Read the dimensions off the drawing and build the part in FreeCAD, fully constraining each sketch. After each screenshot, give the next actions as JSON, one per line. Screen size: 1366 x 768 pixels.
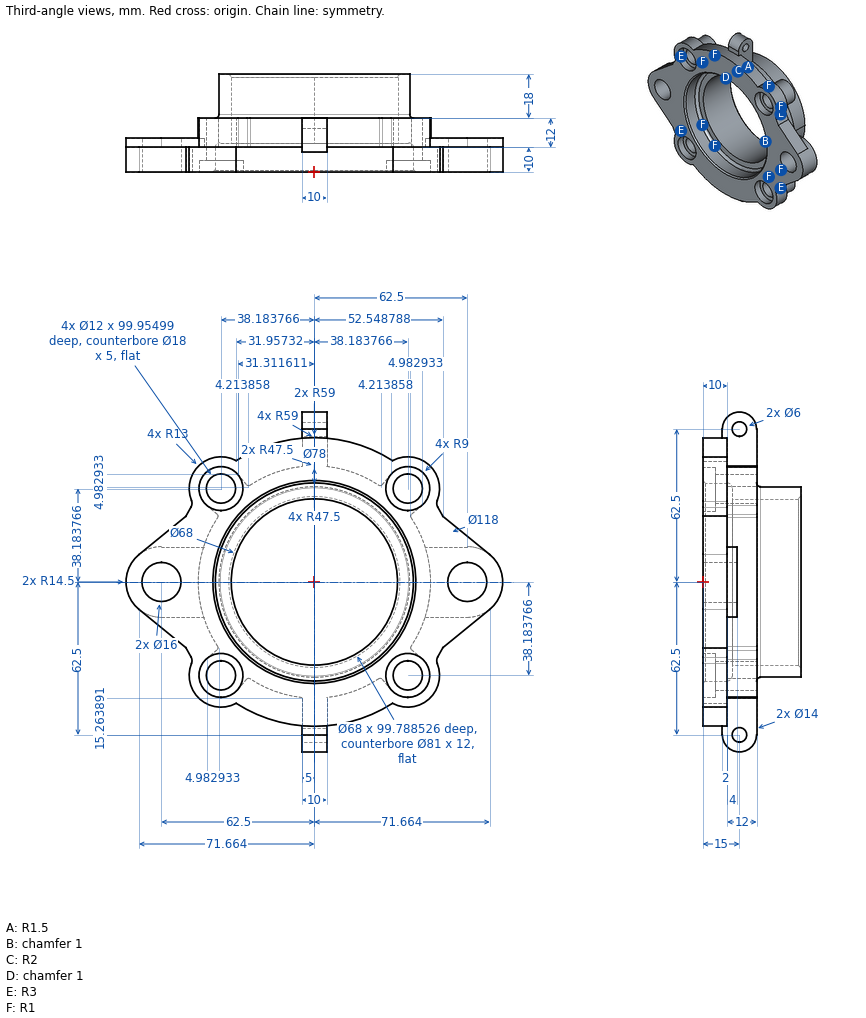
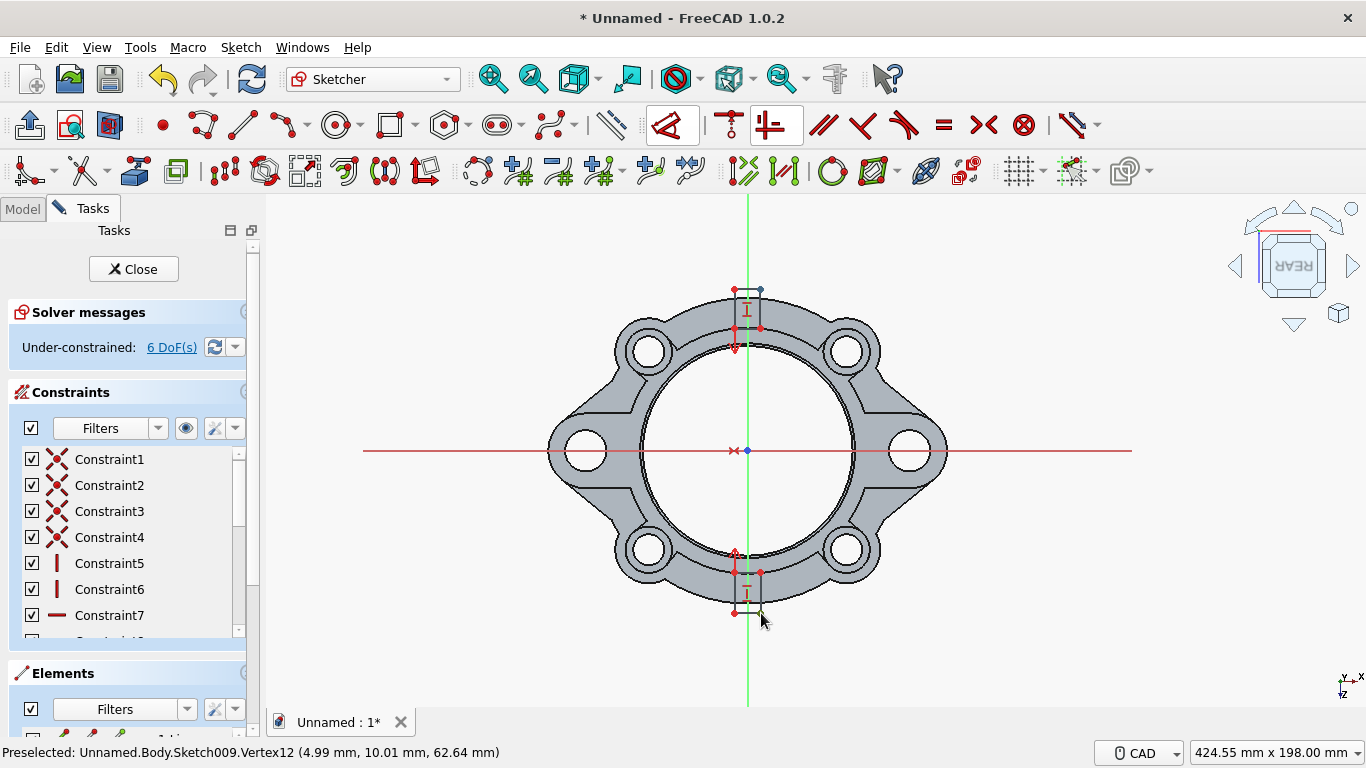
{"action": "left_click", "coordinate": [359, 451]}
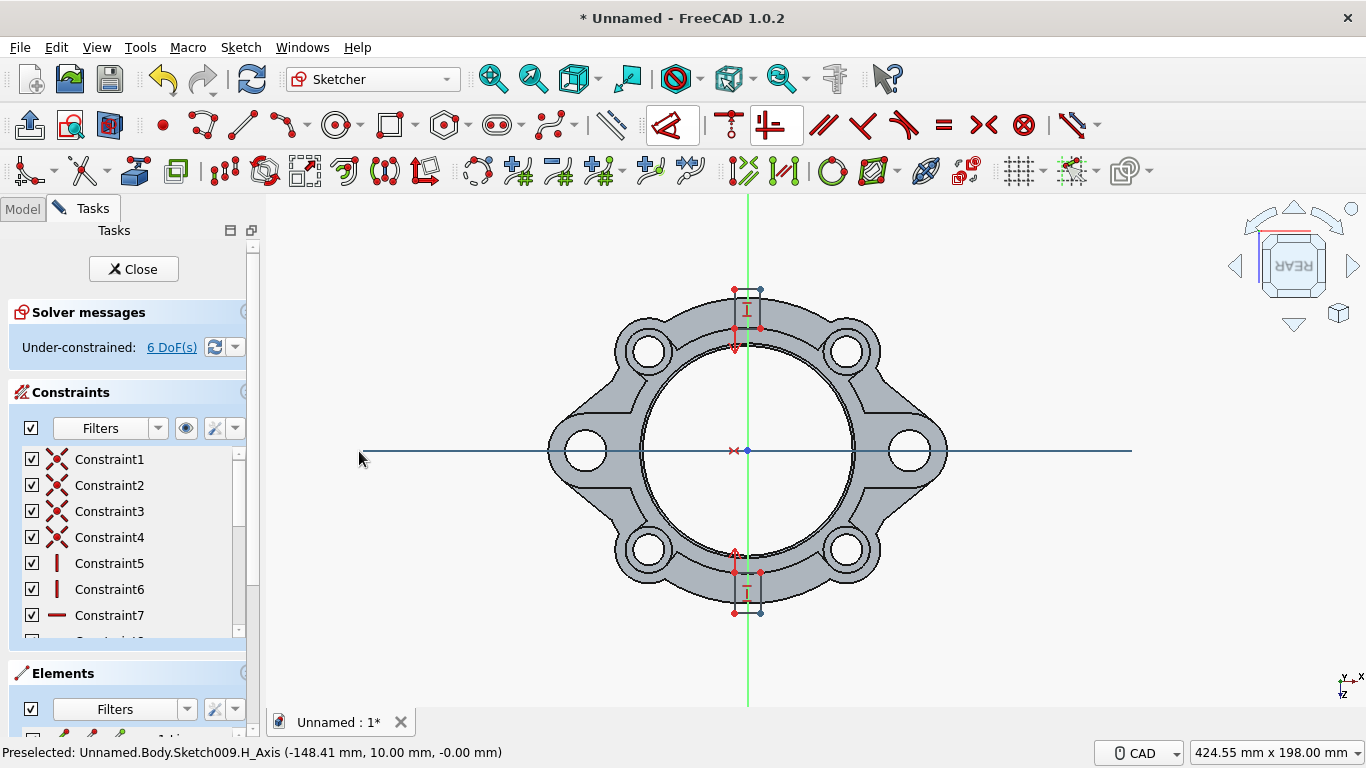
{"action": "left_click", "coordinate": [984, 126]}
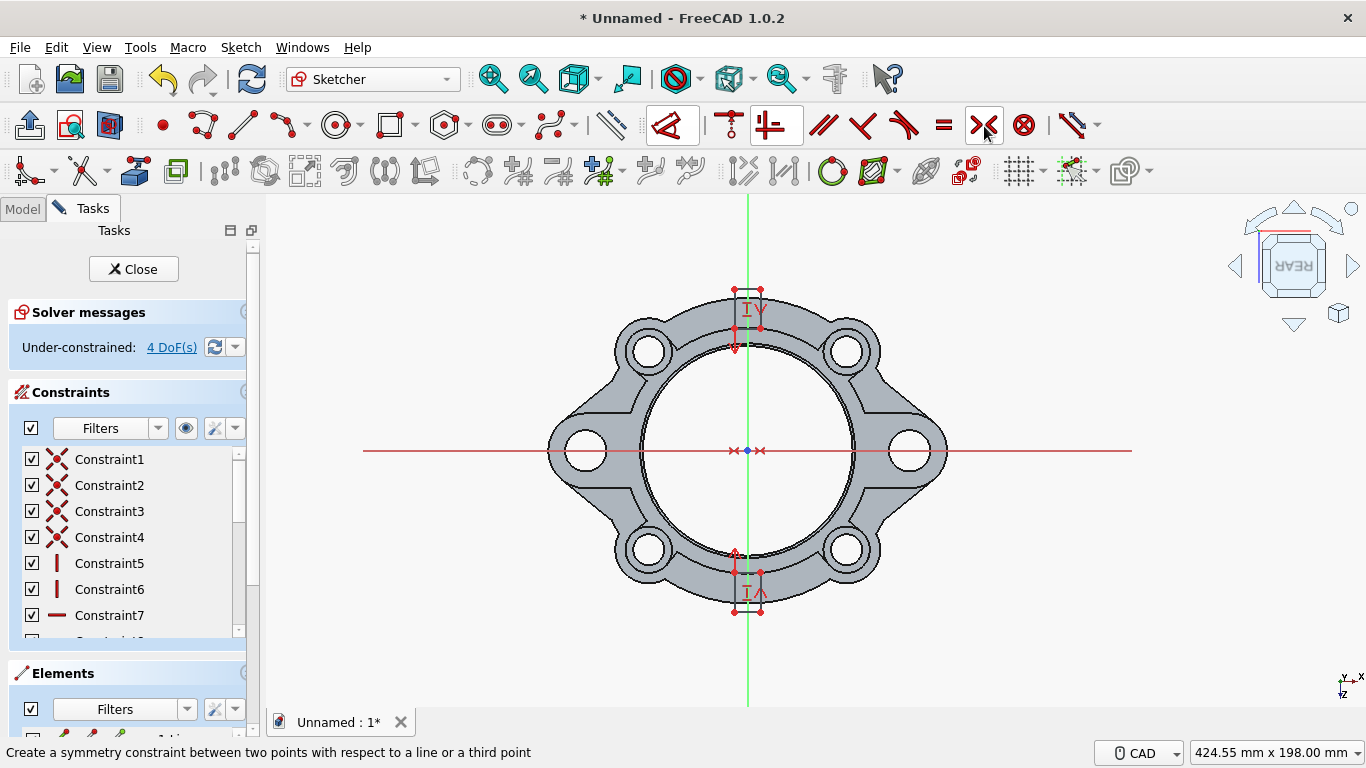
{"action": "scroll", "coordinate": [745, 329], "scroll_direction": "up", "scroll_amount": 3}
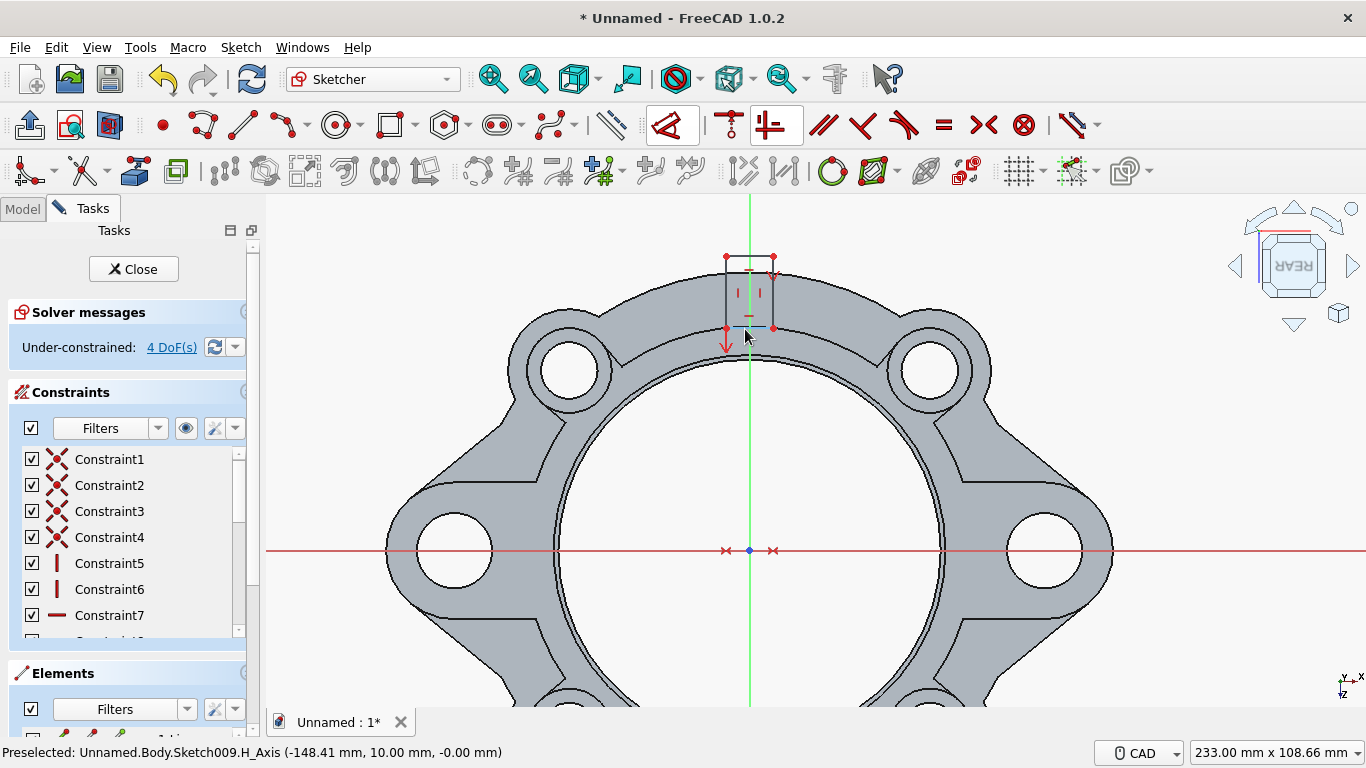
{"action": "left_click", "coordinate": [745, 328]}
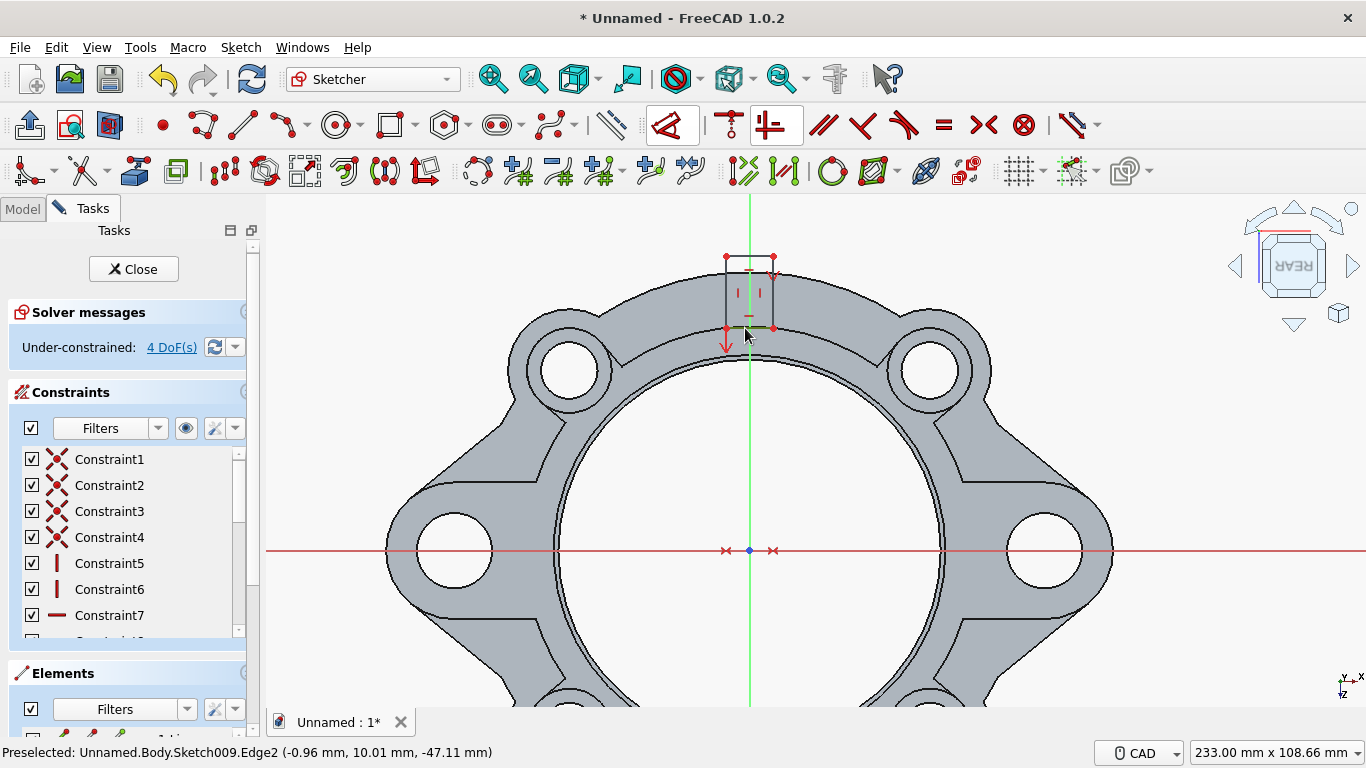
{"action": "key", "text": "l"}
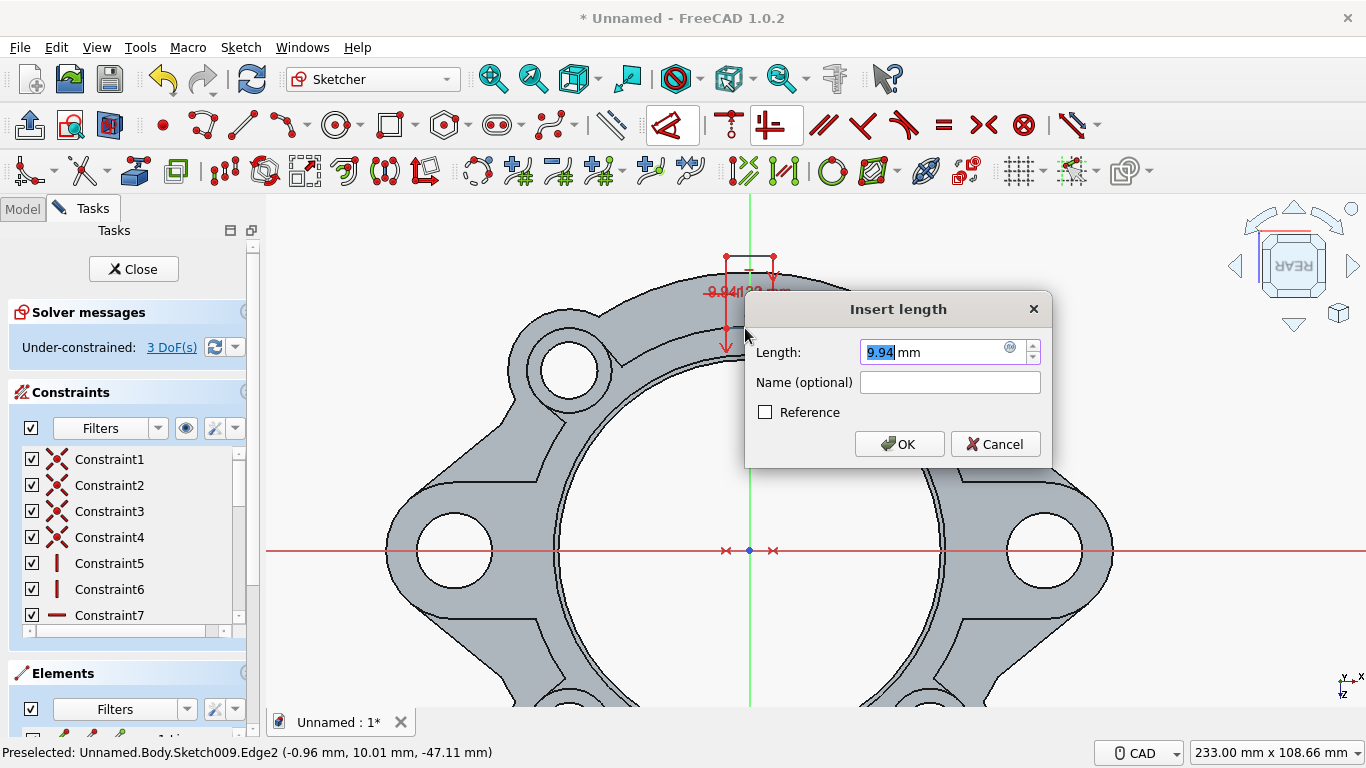
{"action": "type", "text": "10"}
{"action": "key", "text": "Return"}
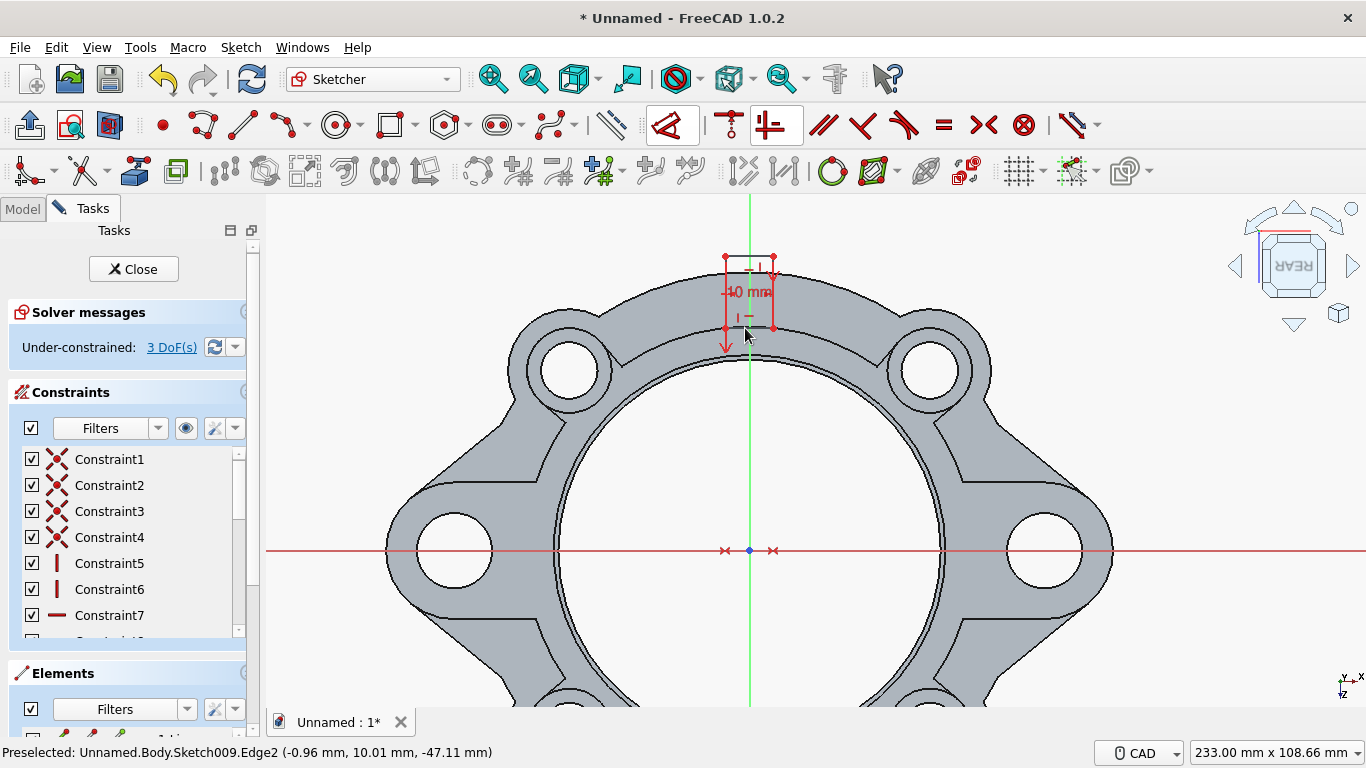
{"action": "scroll", "coordinate": [726, 256], "scroll_direction": "up", "scroll_amount": 3}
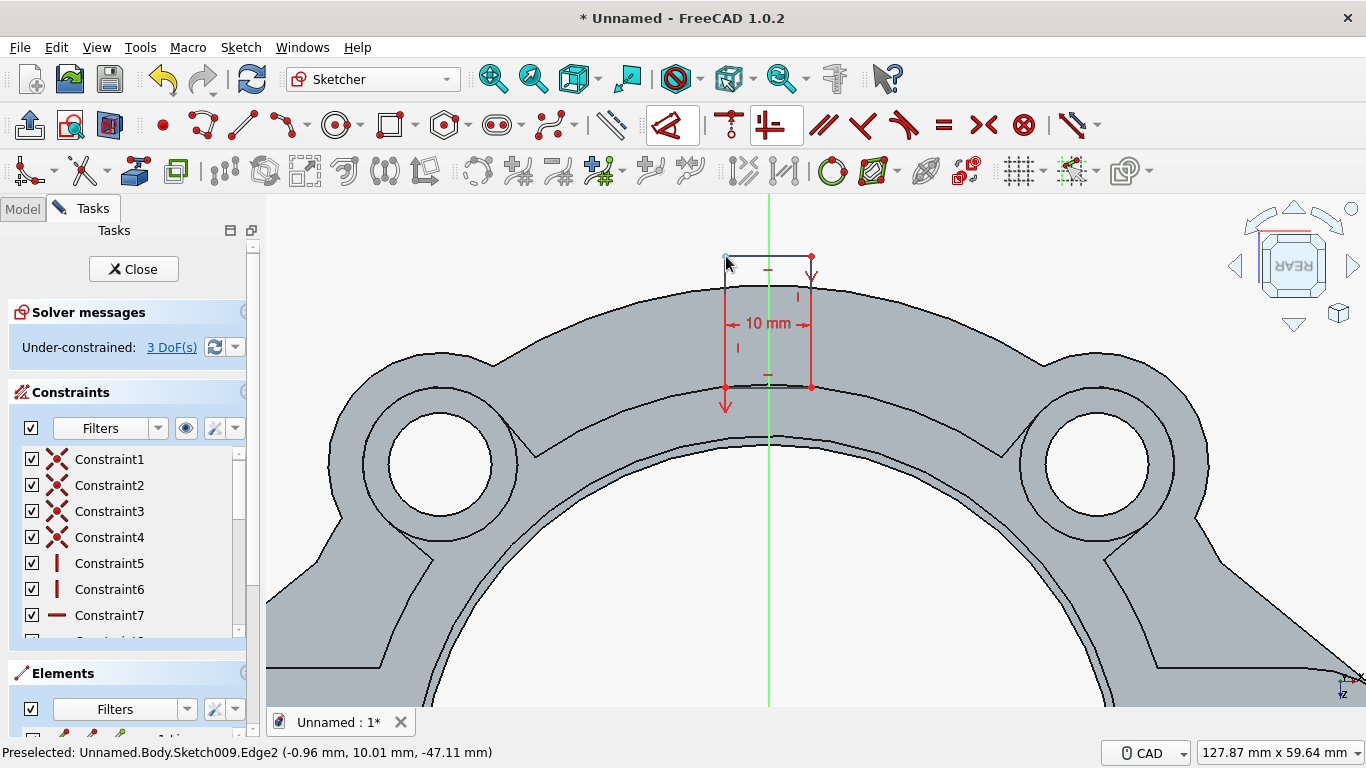
{"action": "left_click", "coordinate": [725, 256]}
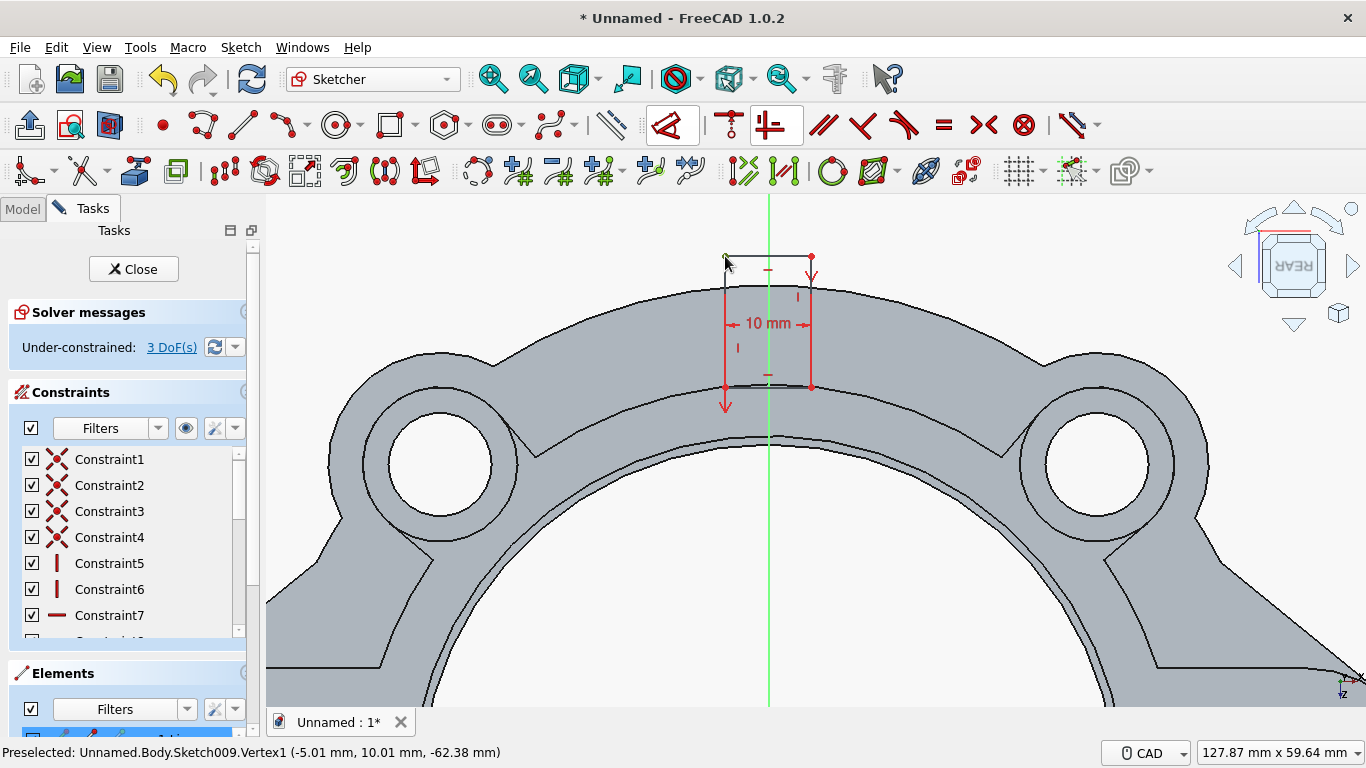
{"action": "key", "text": "l"}